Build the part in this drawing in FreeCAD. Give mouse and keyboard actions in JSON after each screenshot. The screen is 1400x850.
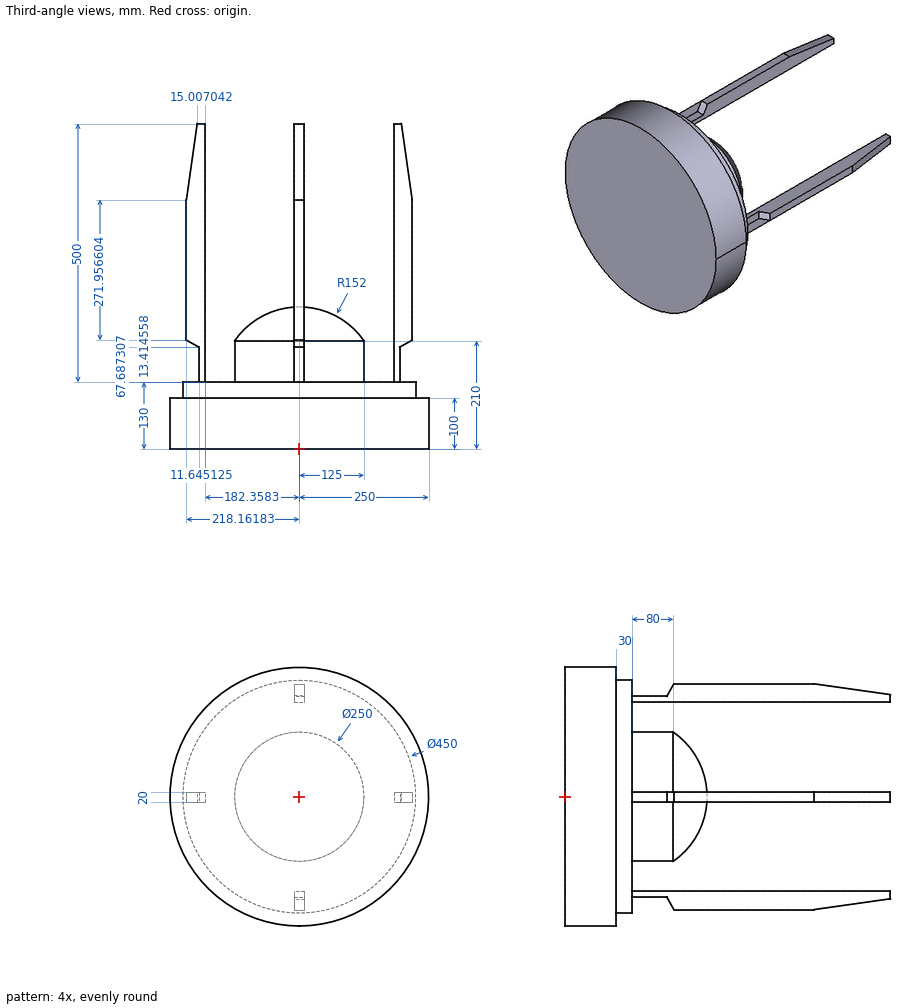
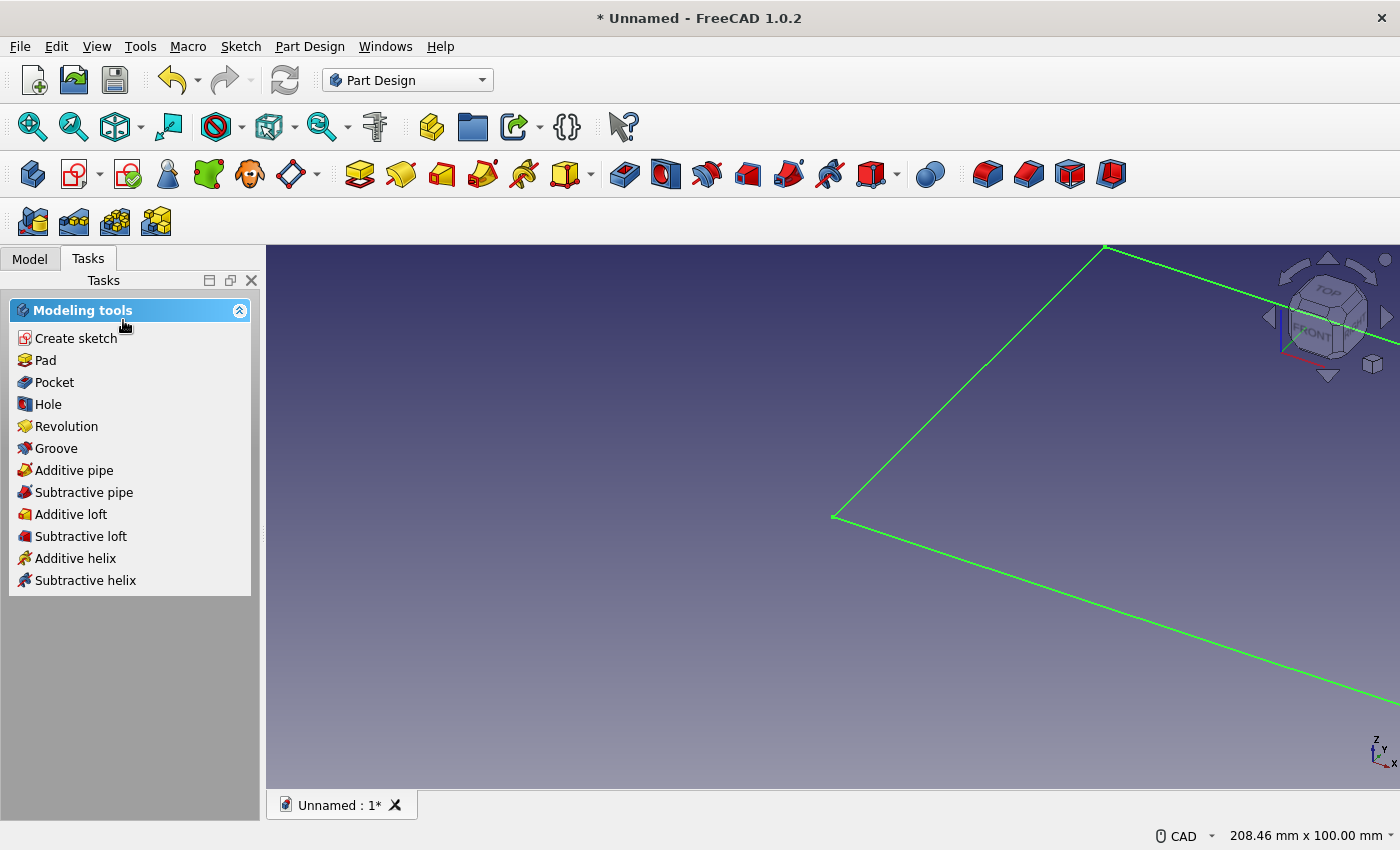
{"action": "left_click", "coordinate": [401, 174]}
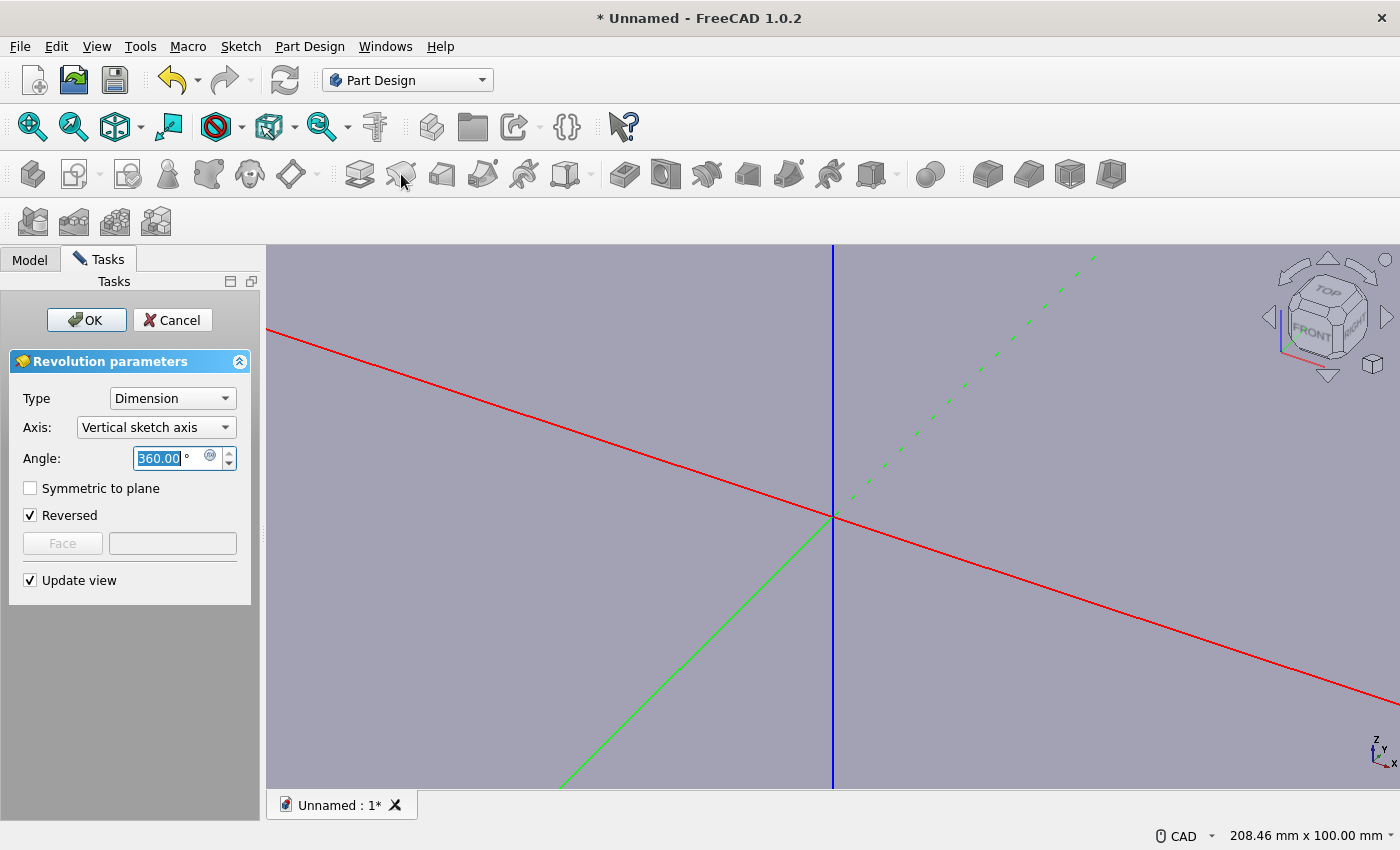
{"action": "left_click", "coordinate": [87, 320]}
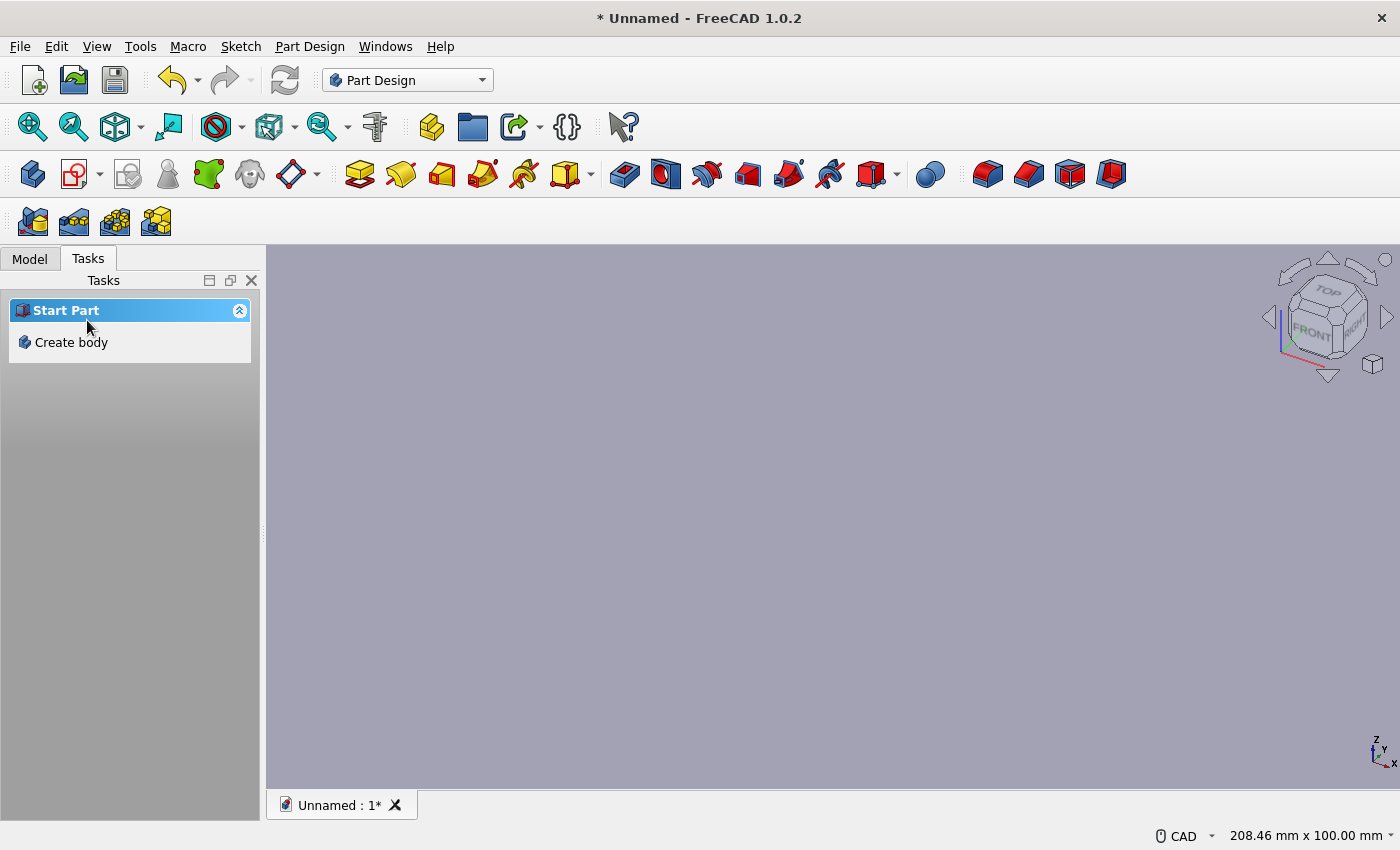
{"action": "left_click", "coordinate": [33, 128]}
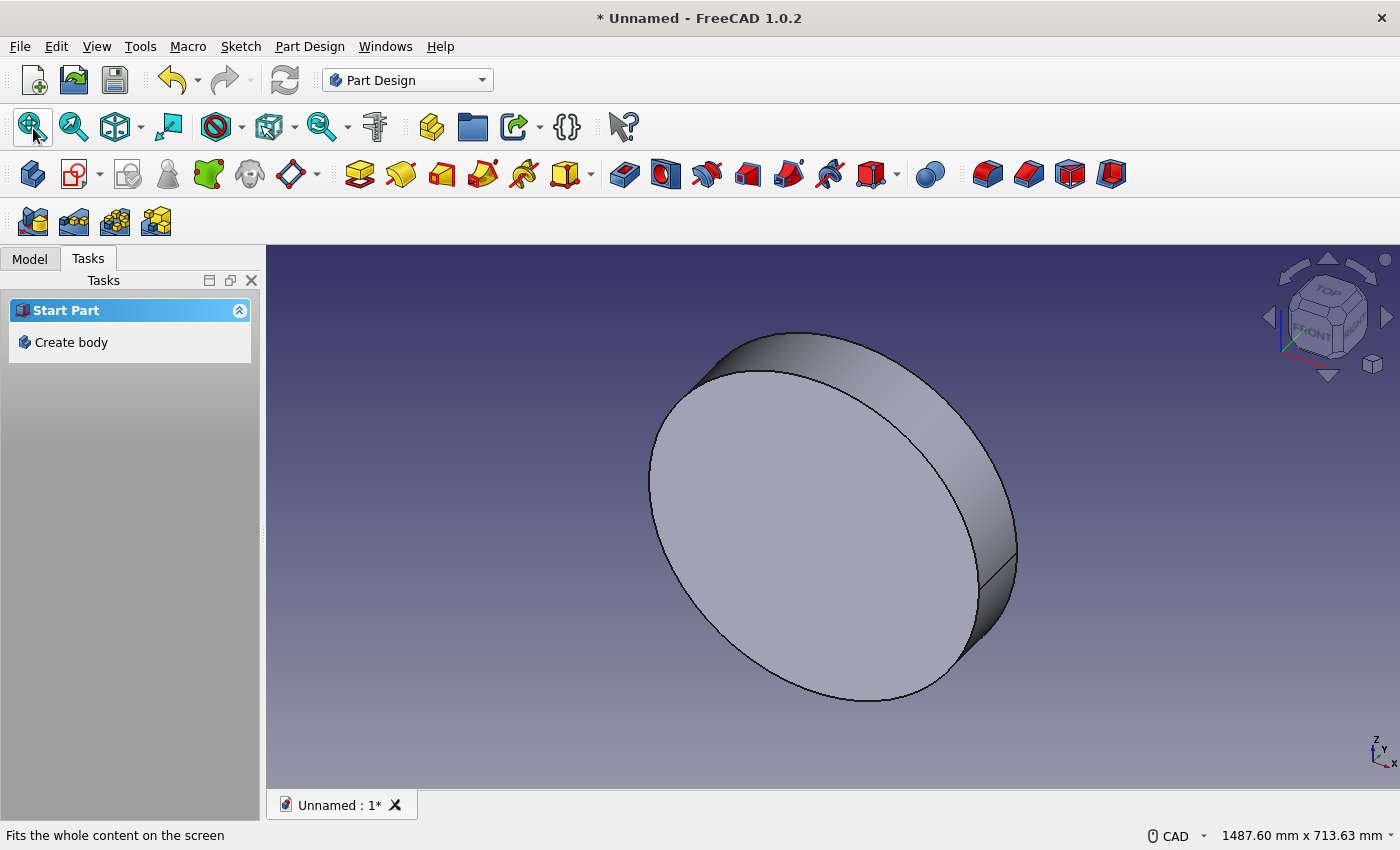
{"action": "key", "text": "4"}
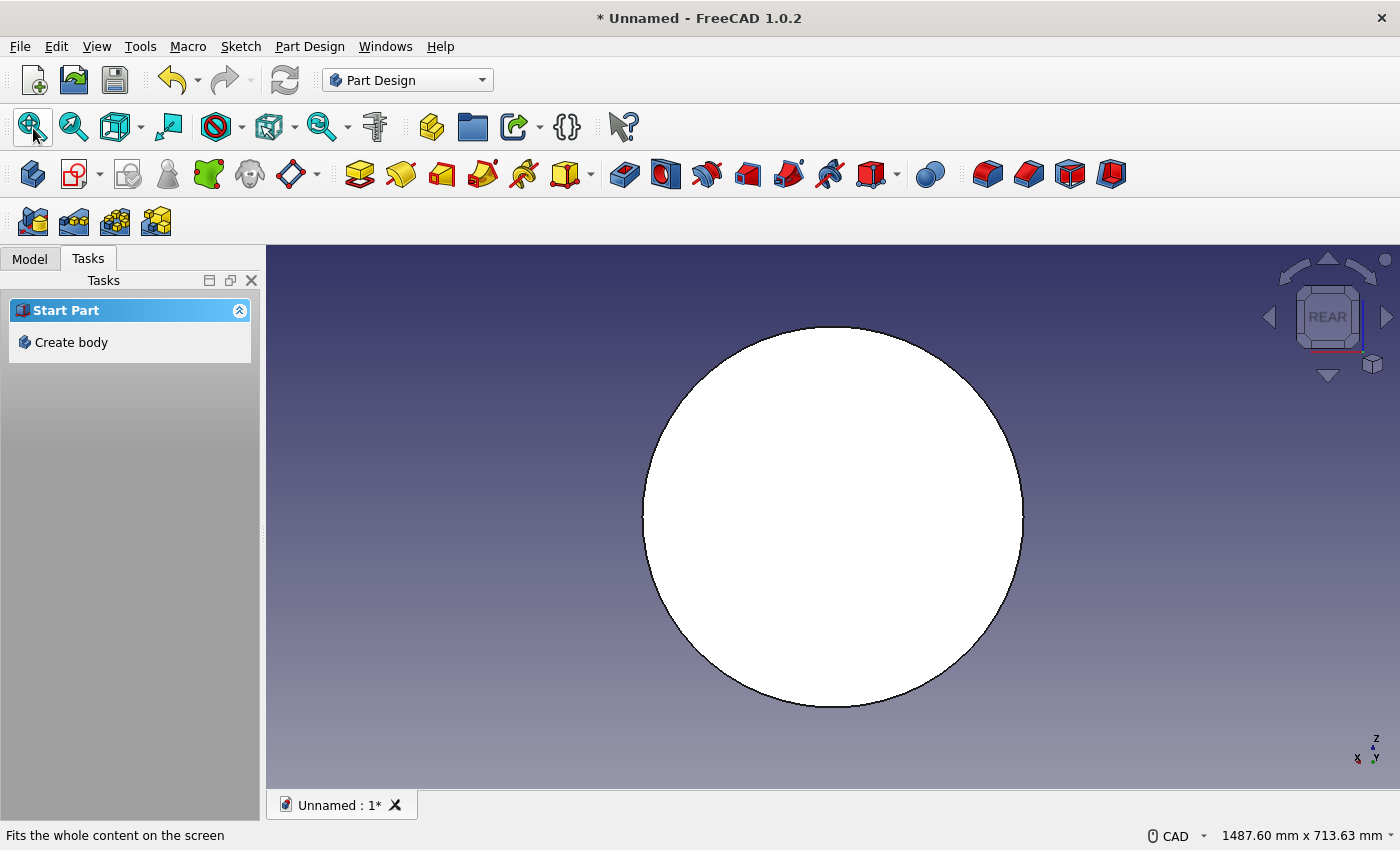
{"action": "left_click", "coordinate": [833, 516]}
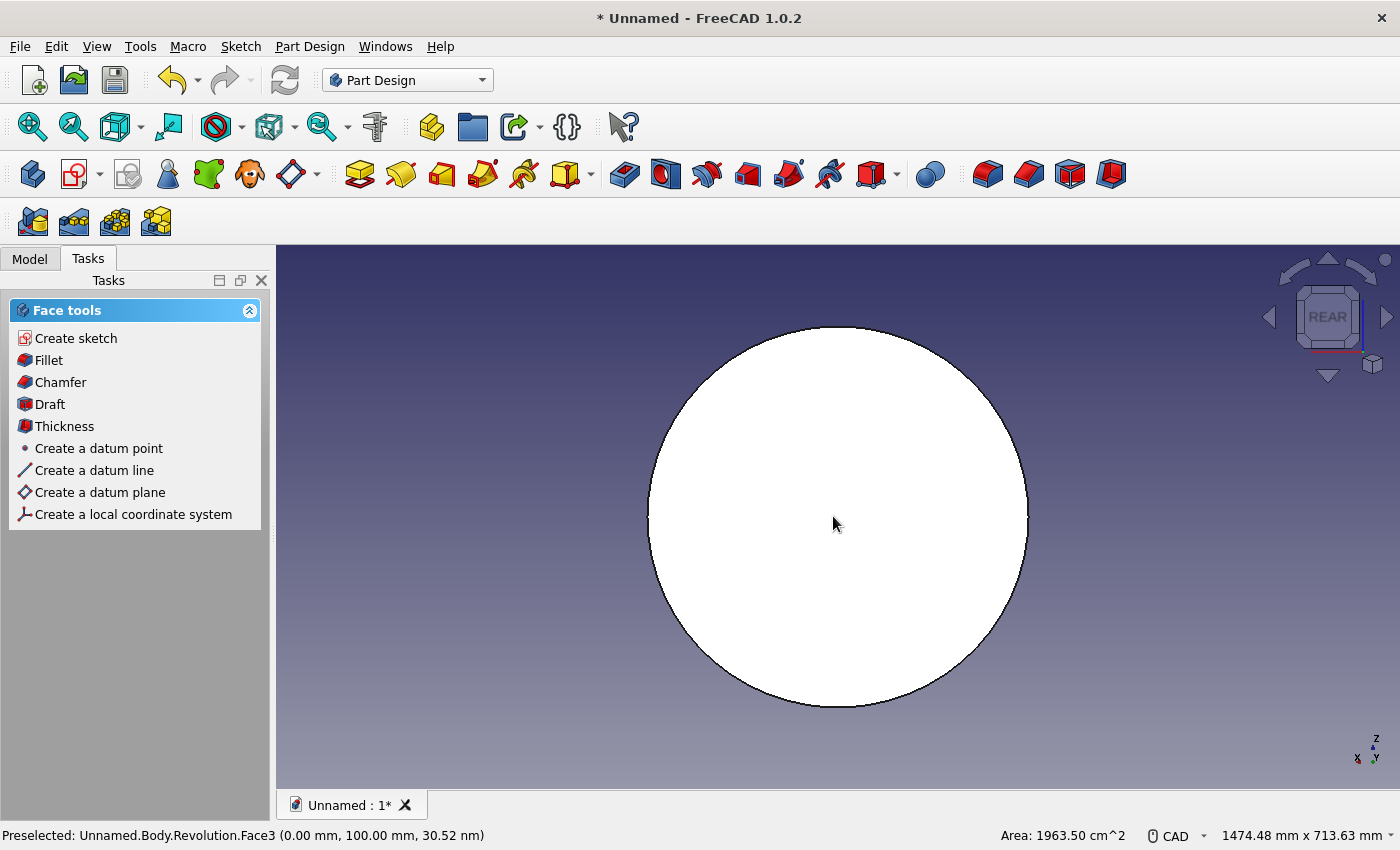
{"action": "left_click", "coordinate": [74, 174]}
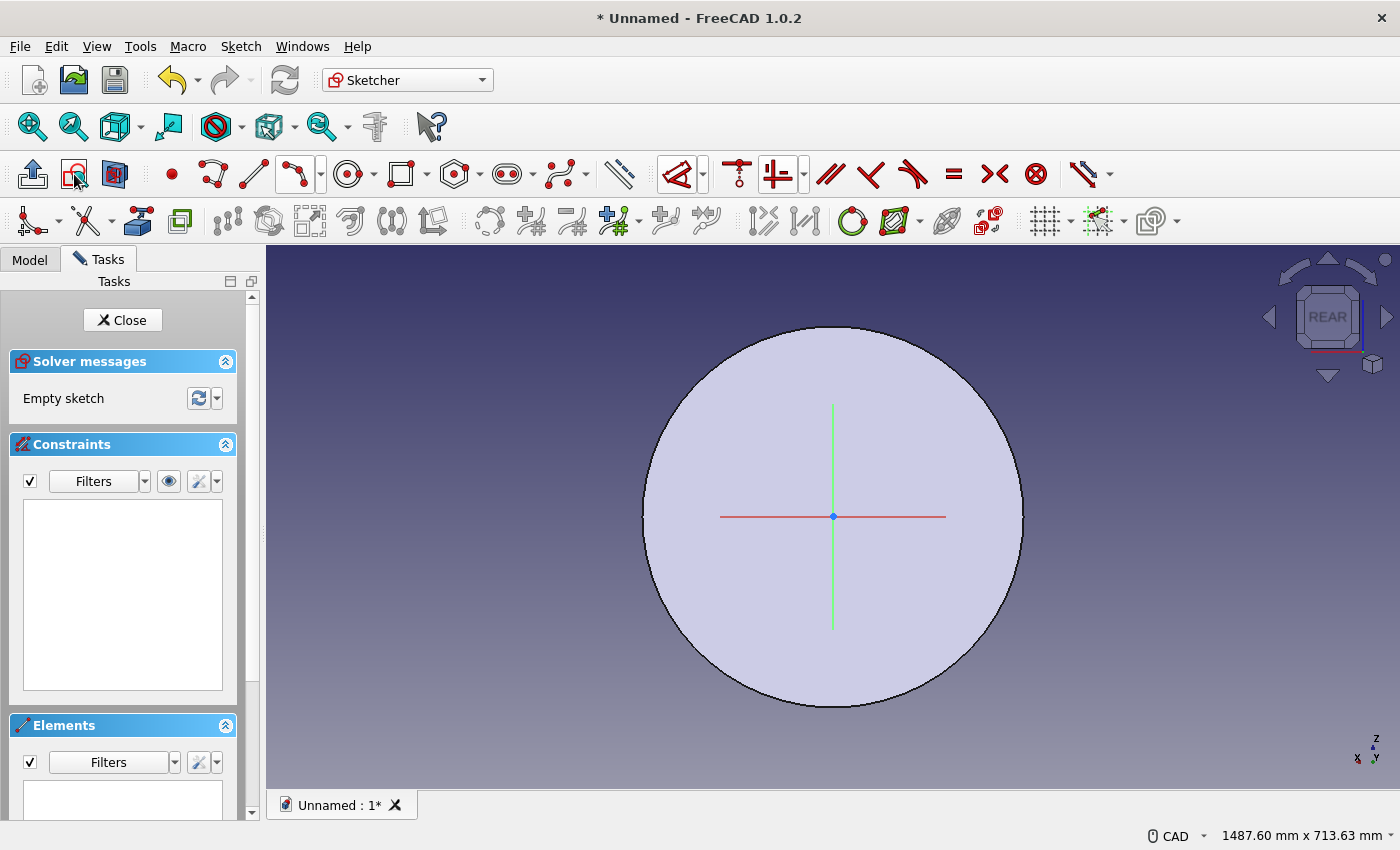
{"action": "left_click", "coordinate": [348, 174]}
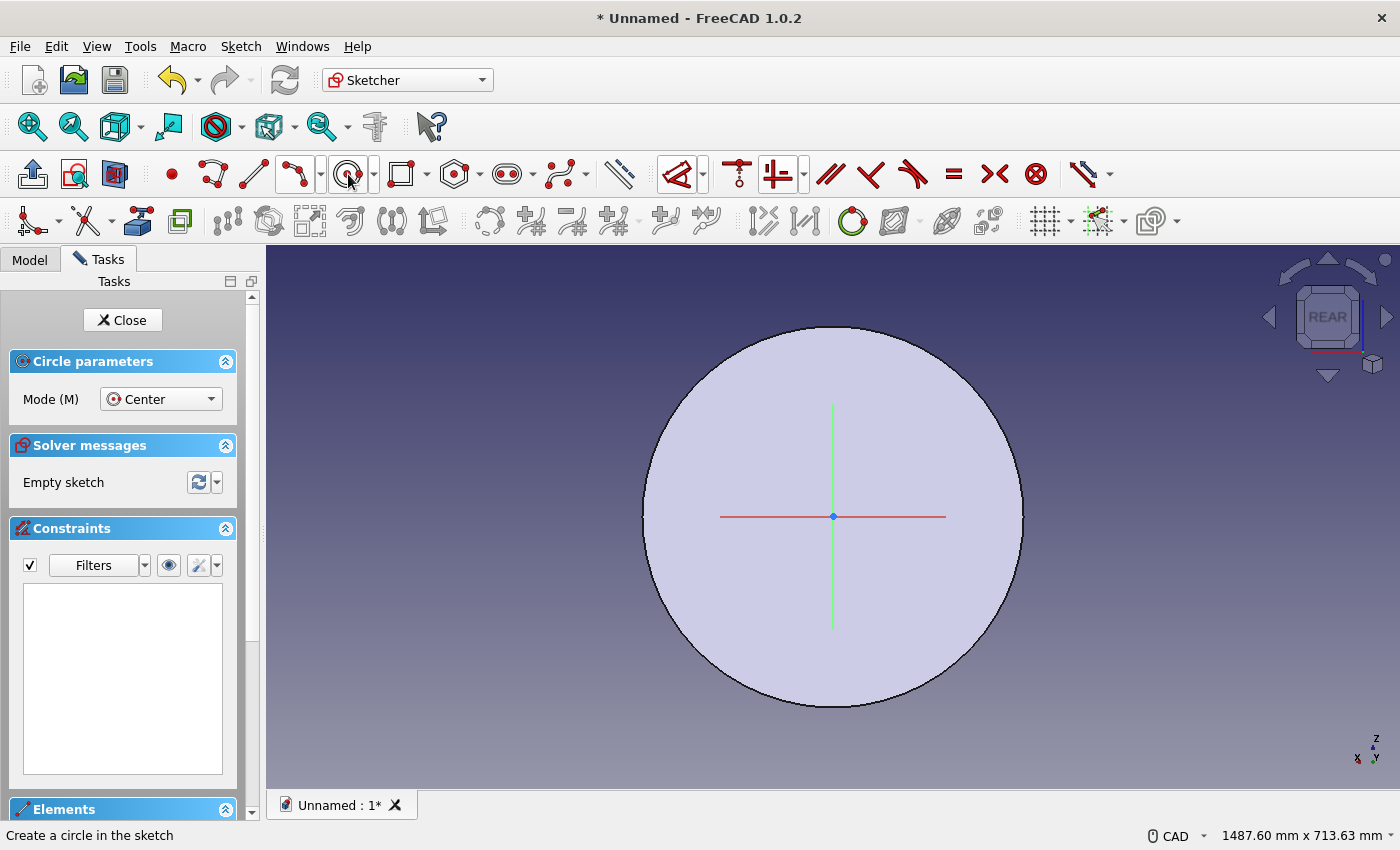
{"action": "left_click", "coordinate": [833, 517]}
{"action": "left_click", "coordinate": [954, 396]}
{"action": "key", "text": "Escape"}